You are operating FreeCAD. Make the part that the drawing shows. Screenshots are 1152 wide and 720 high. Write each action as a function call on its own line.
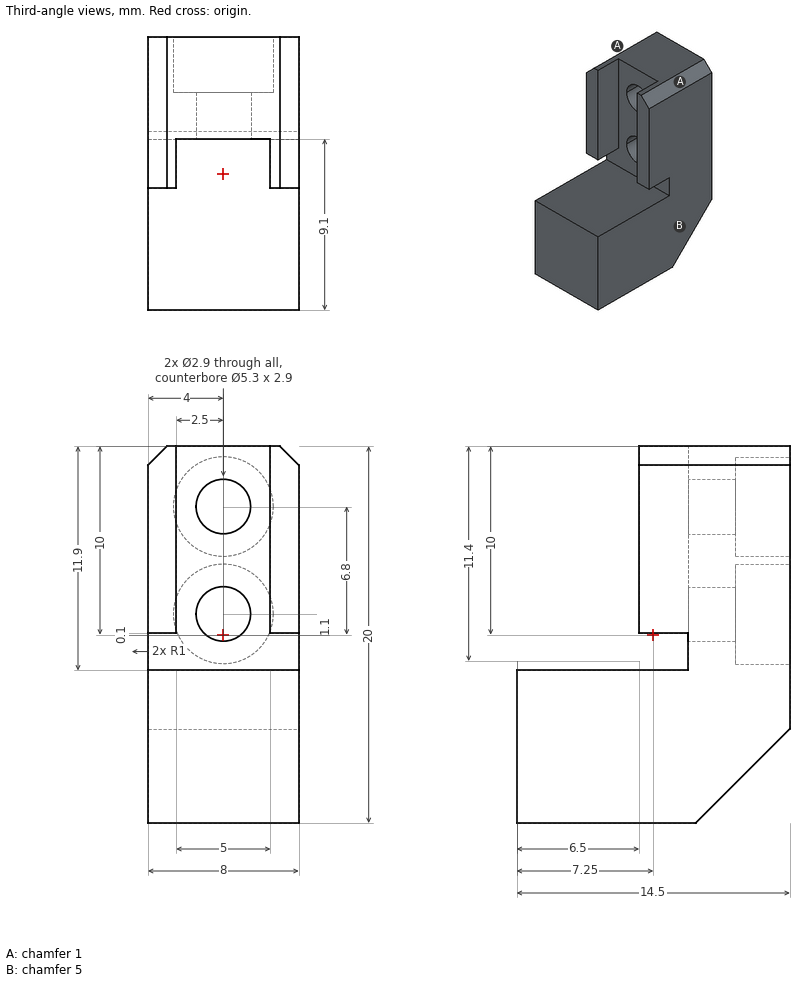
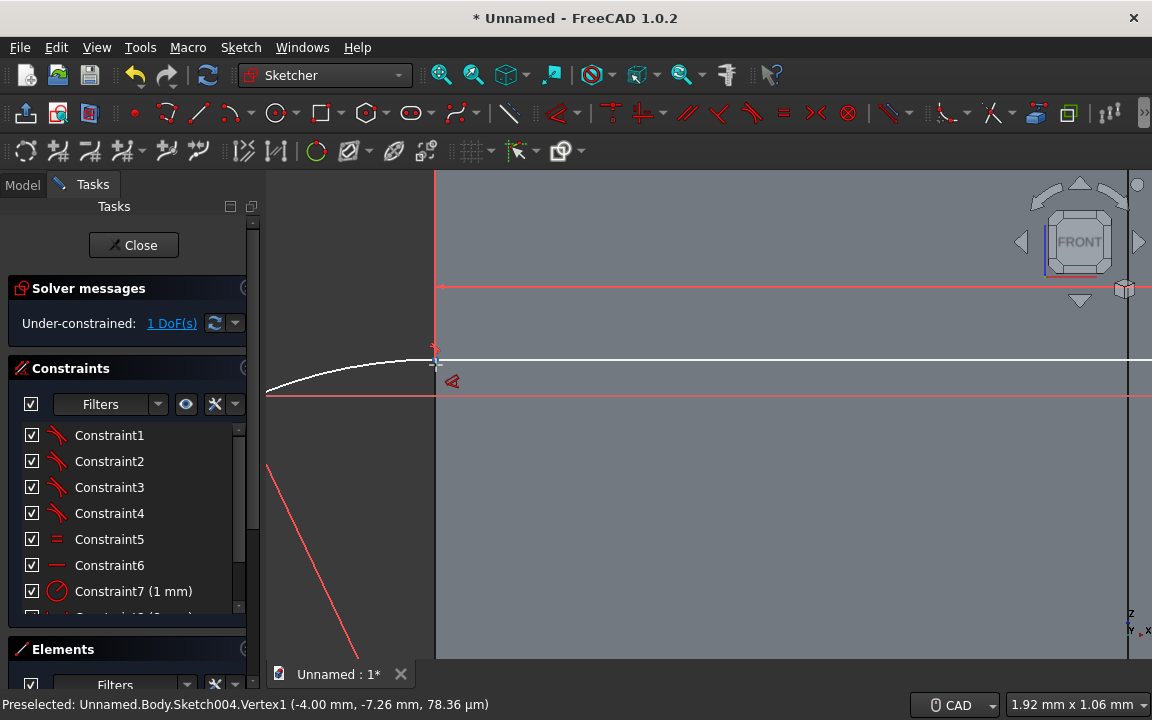
click(435, 360)
click(401, 378)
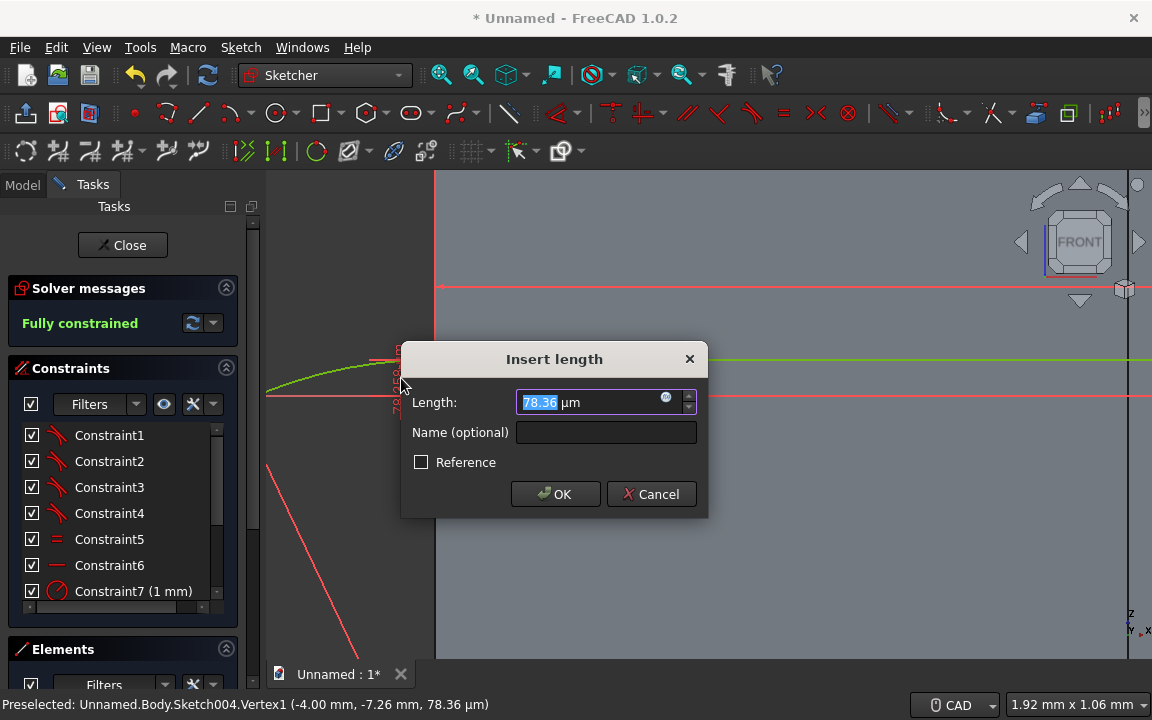
key(ctrl+a)
text(0.1 mm)
key(Return)
key(Escape)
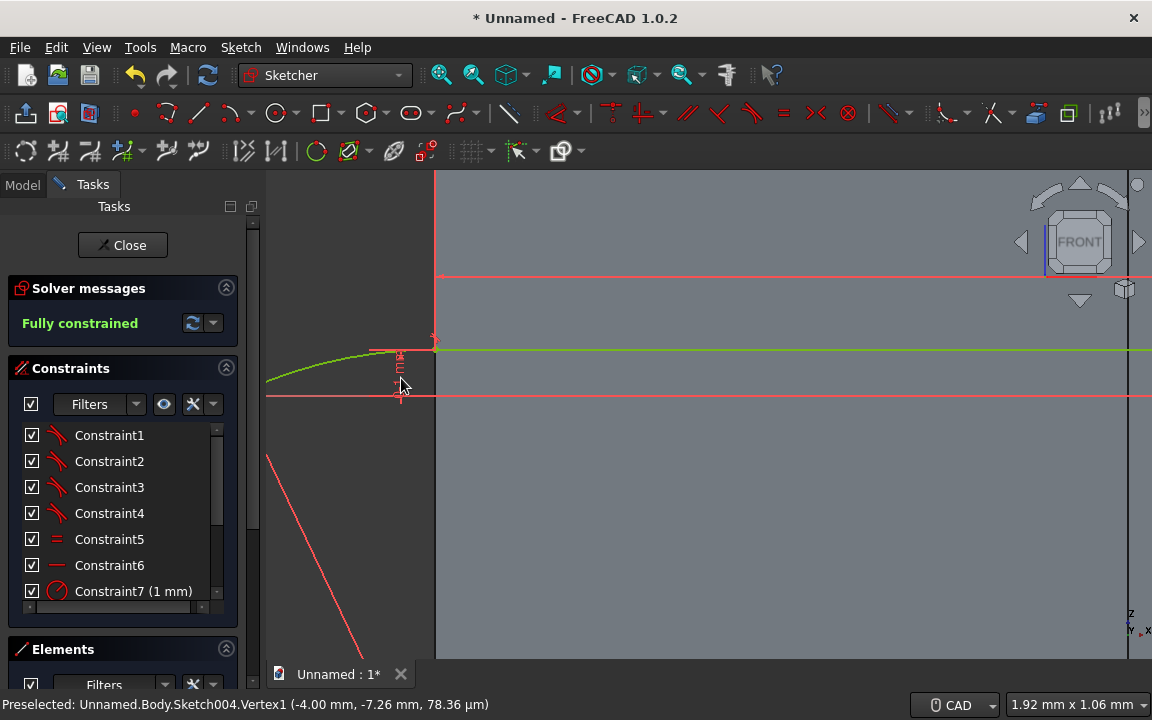
click(123, 245)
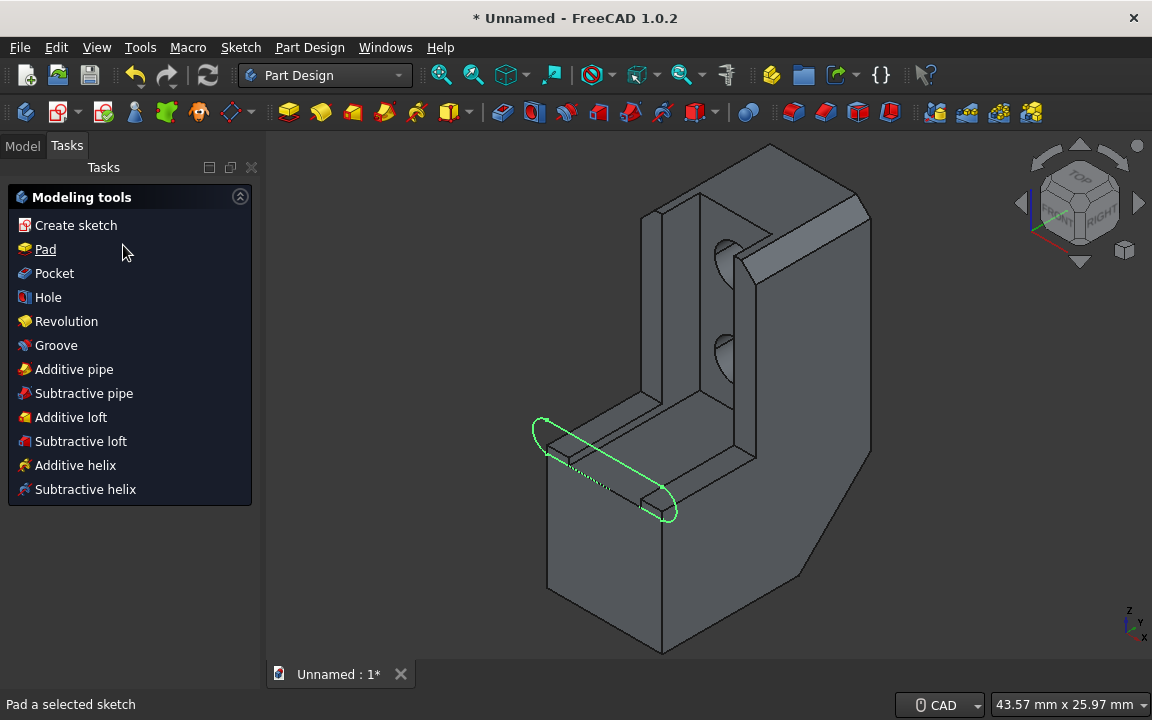
click(504, 112)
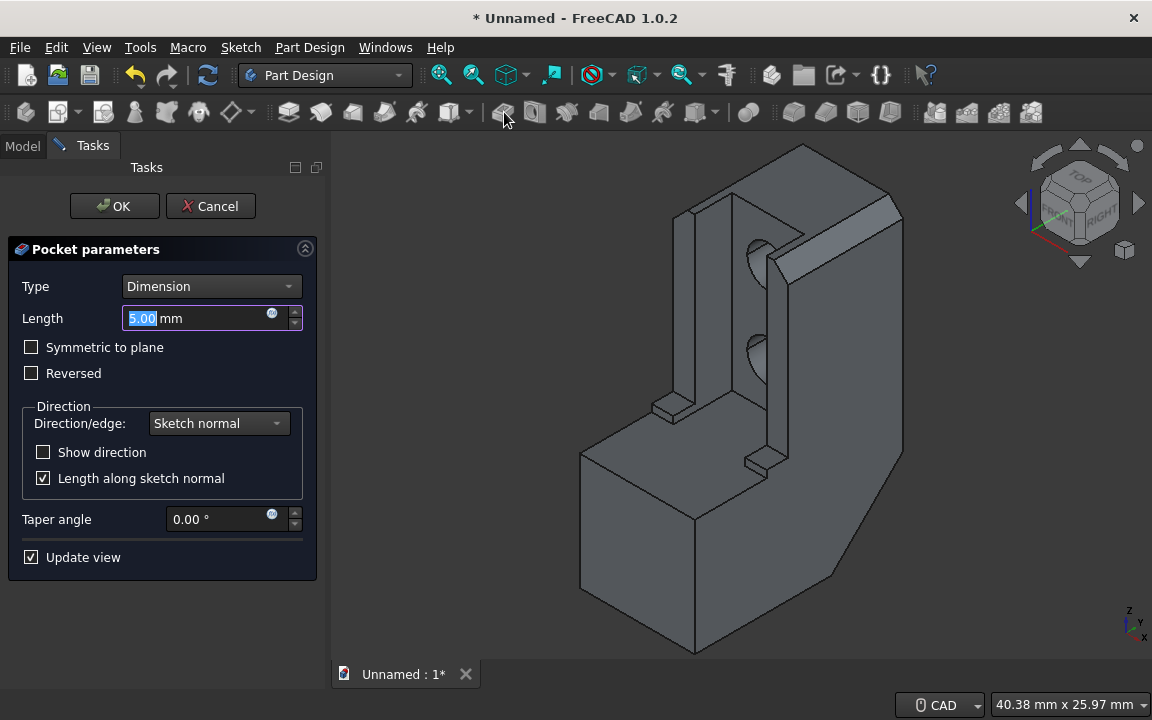
text(9.1)
key(Tab)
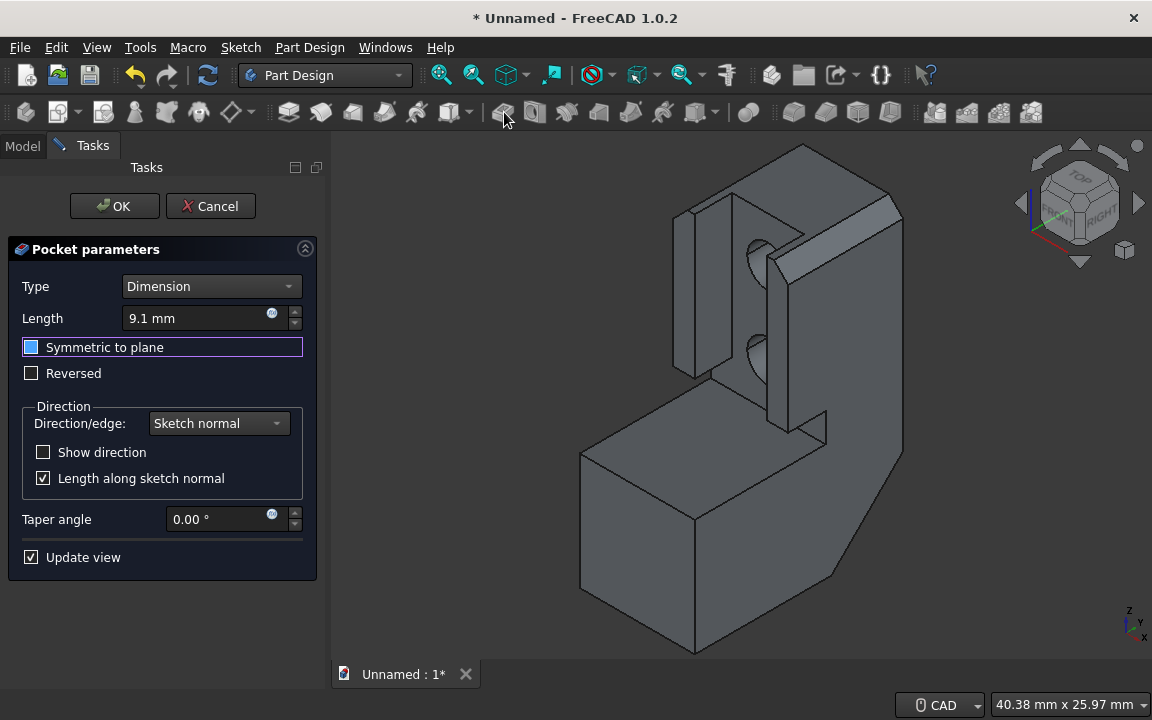
click(115, 206)